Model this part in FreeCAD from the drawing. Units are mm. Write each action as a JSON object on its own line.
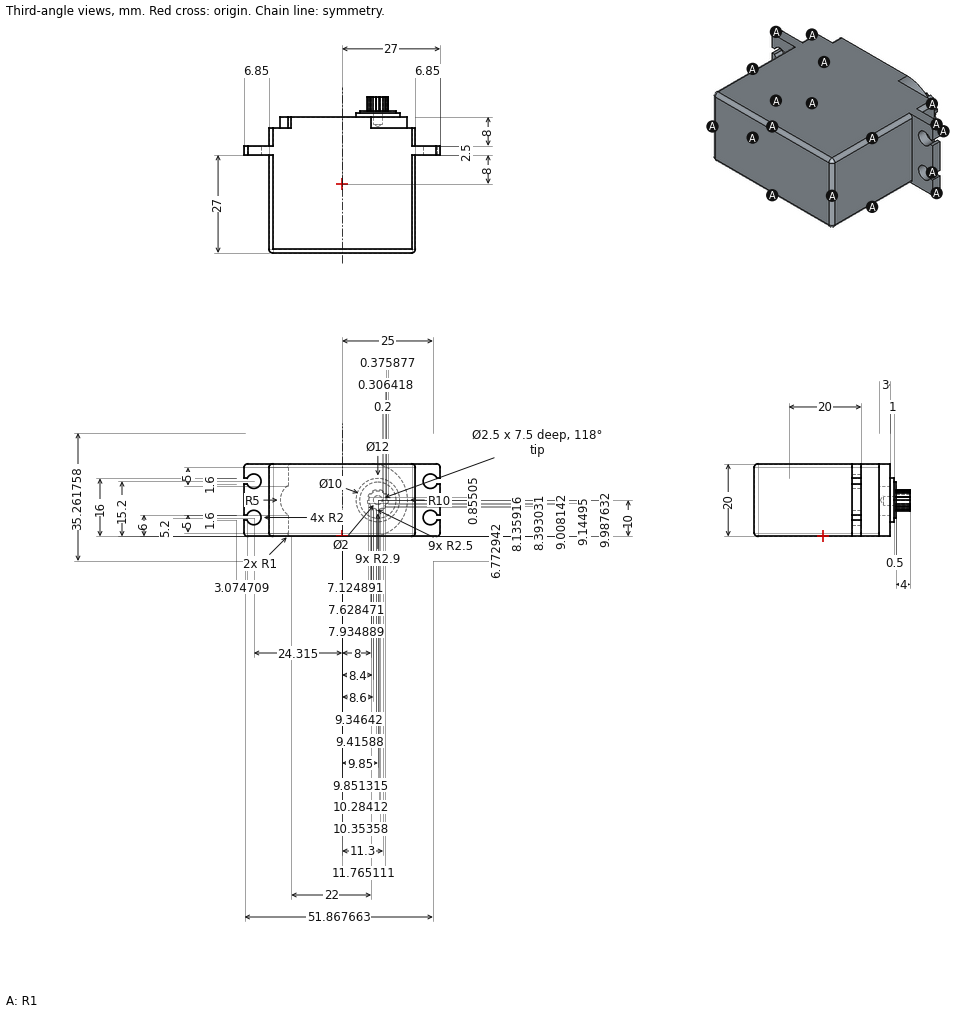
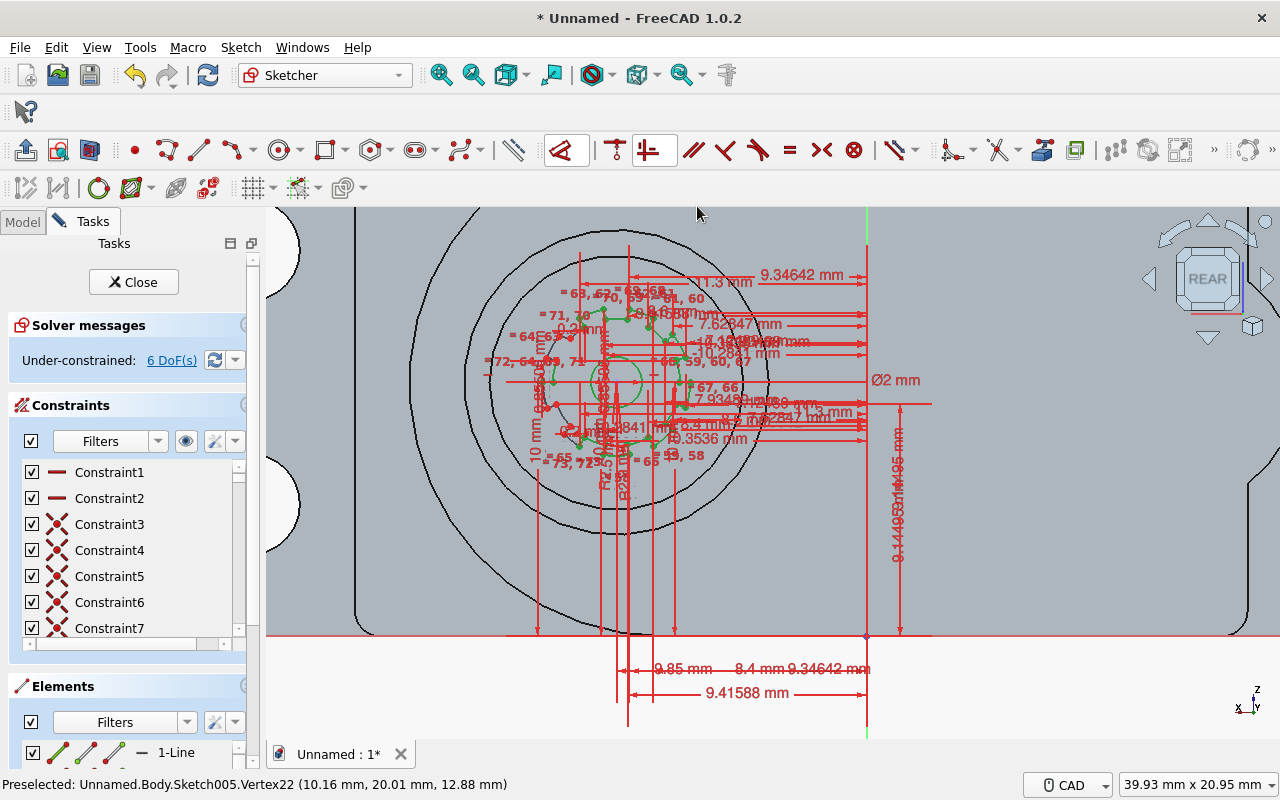
{"action": "left_click", "coordinate": [548, 408]}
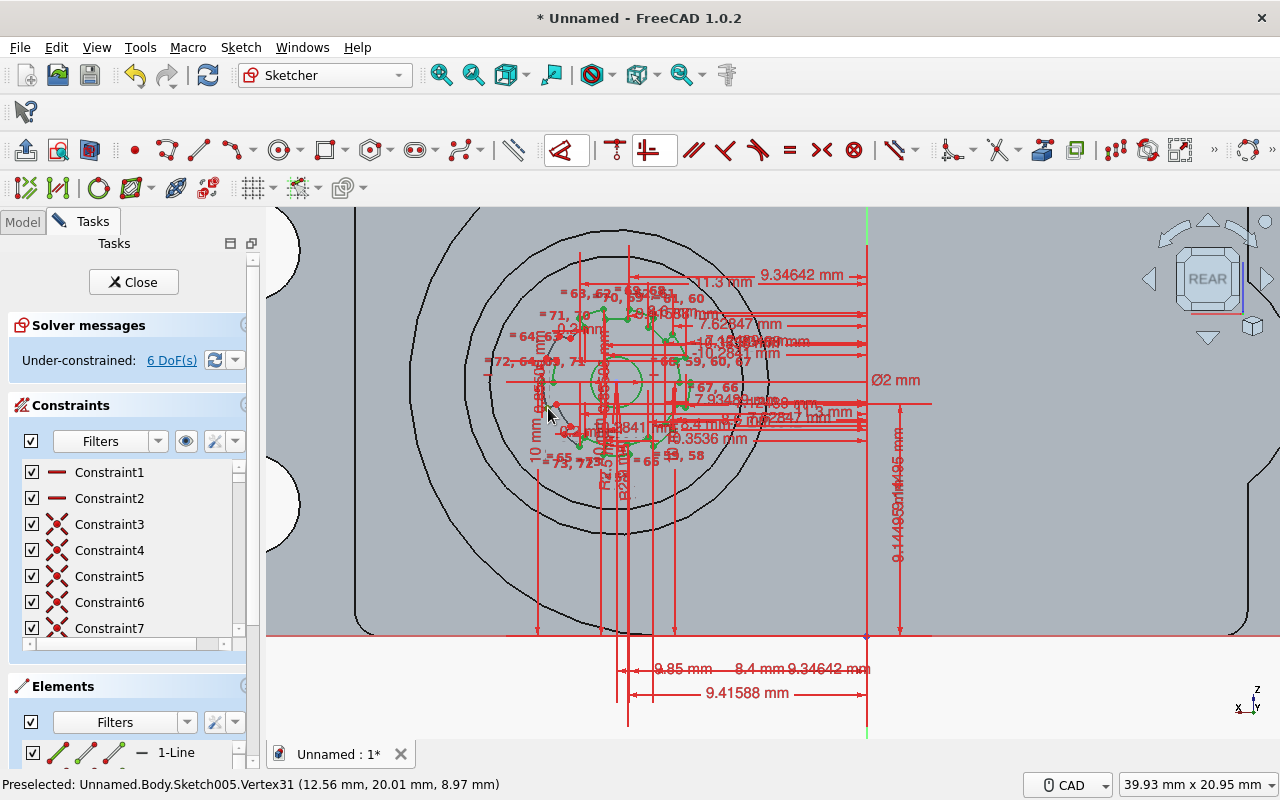
{"action": "left_click", "coordinate": [584, 150]}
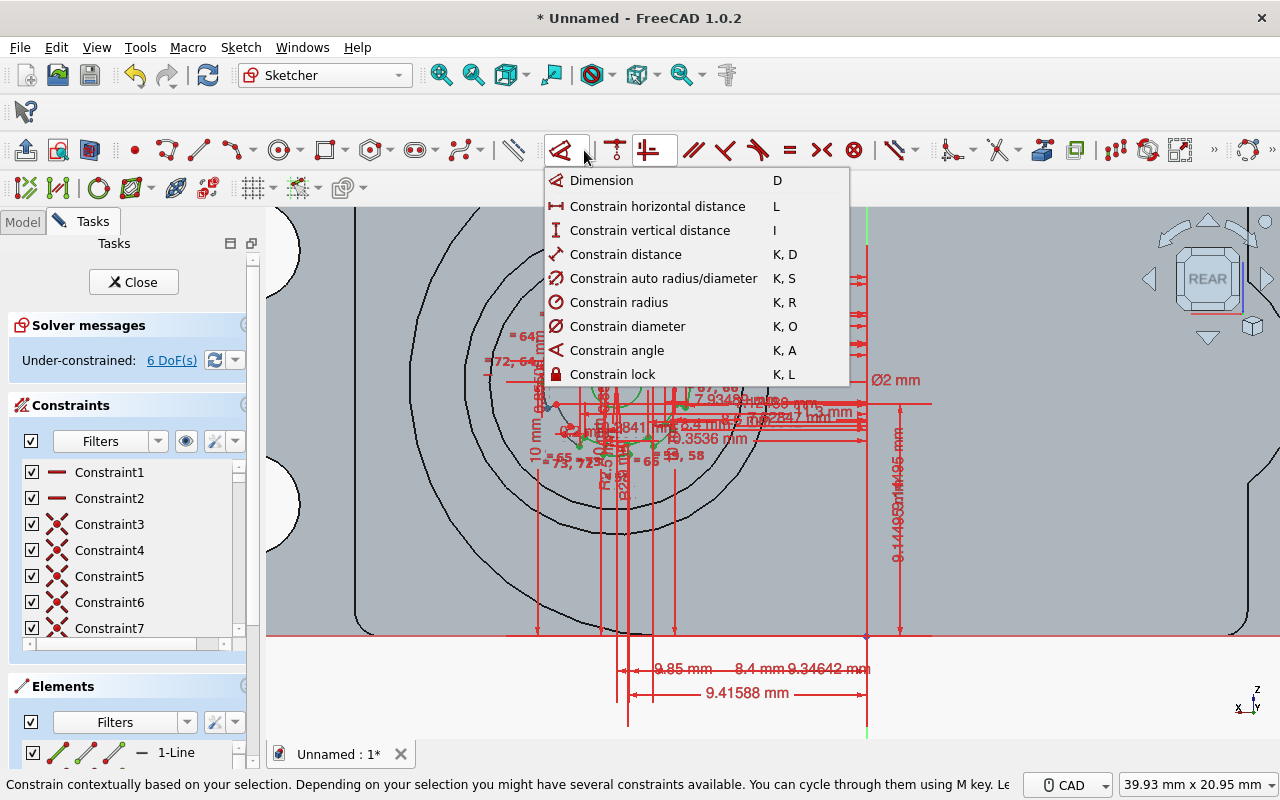
{"action": "left_click", "coordinate": [697, 230]}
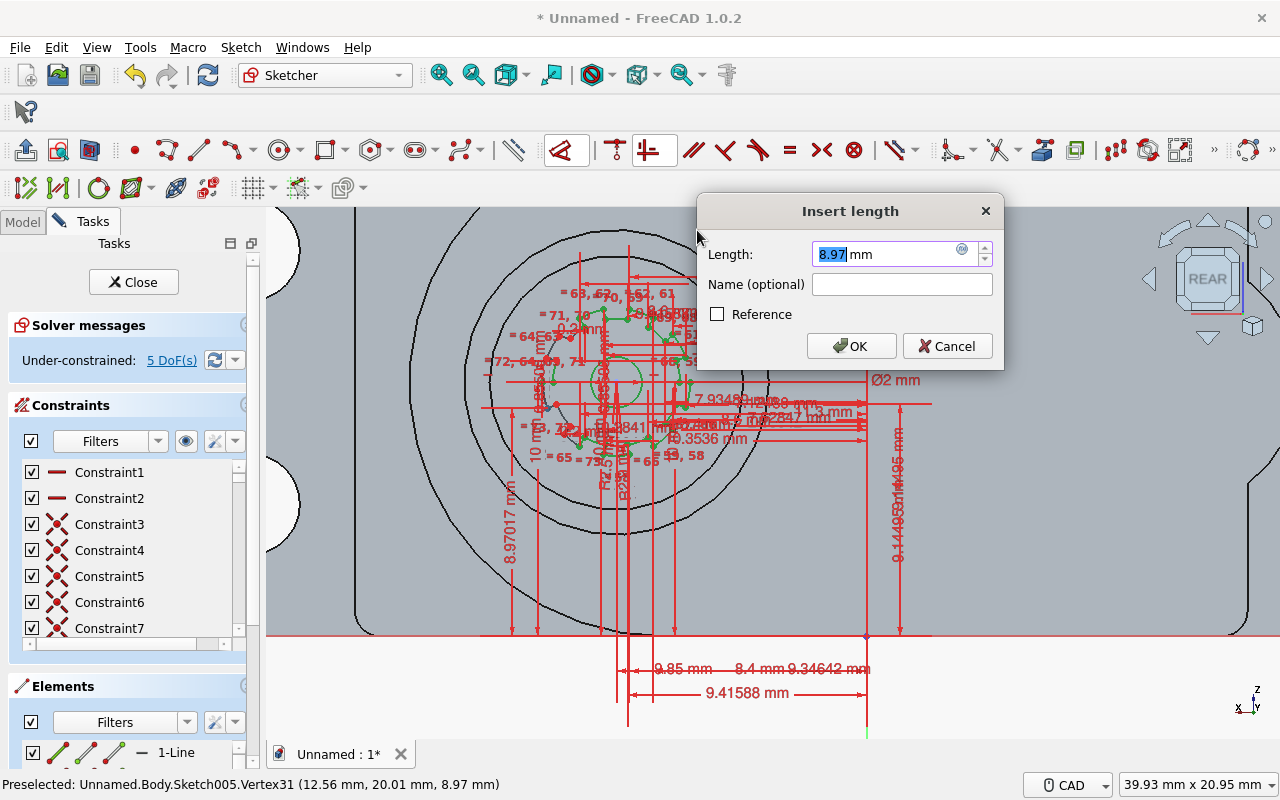
{"action": "type", "text": "9.008142"}
{"action": "key", "text": "Return"}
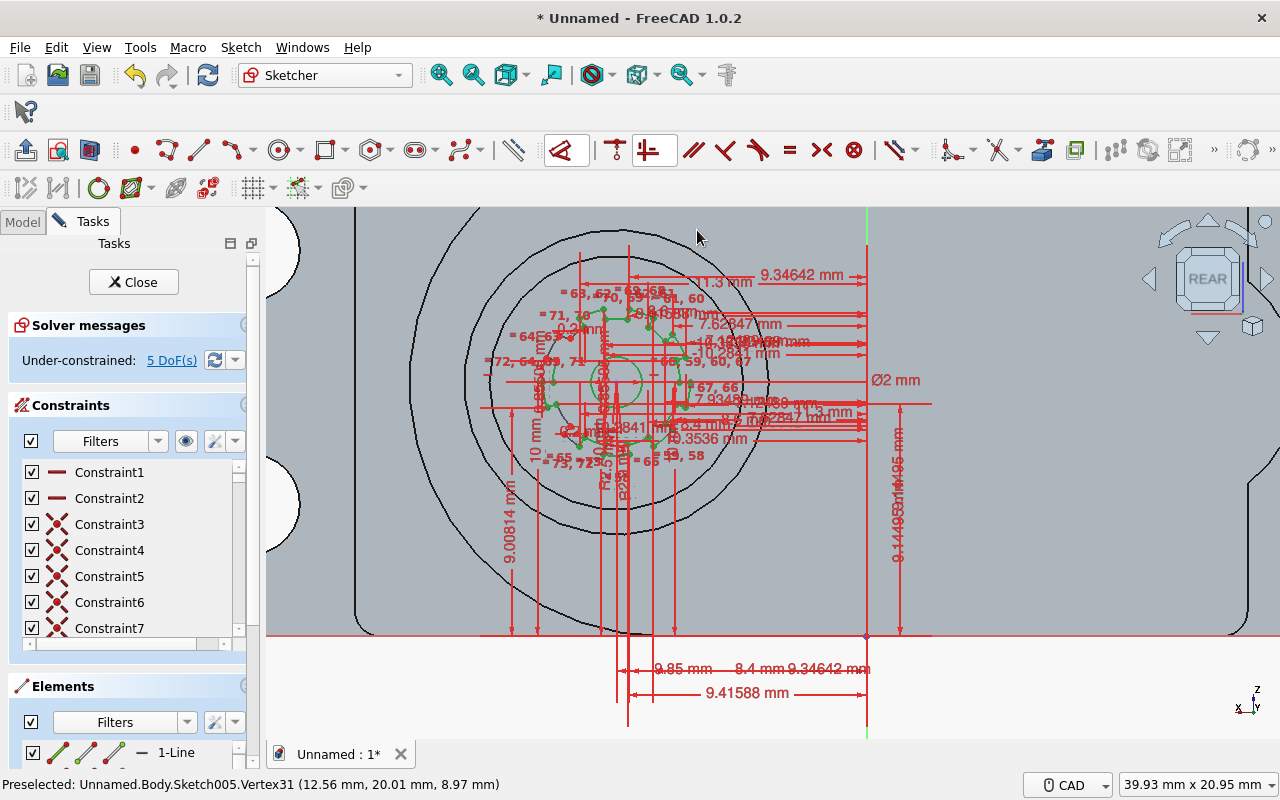
{"action": "left_click", "coordinate": [571, 426]}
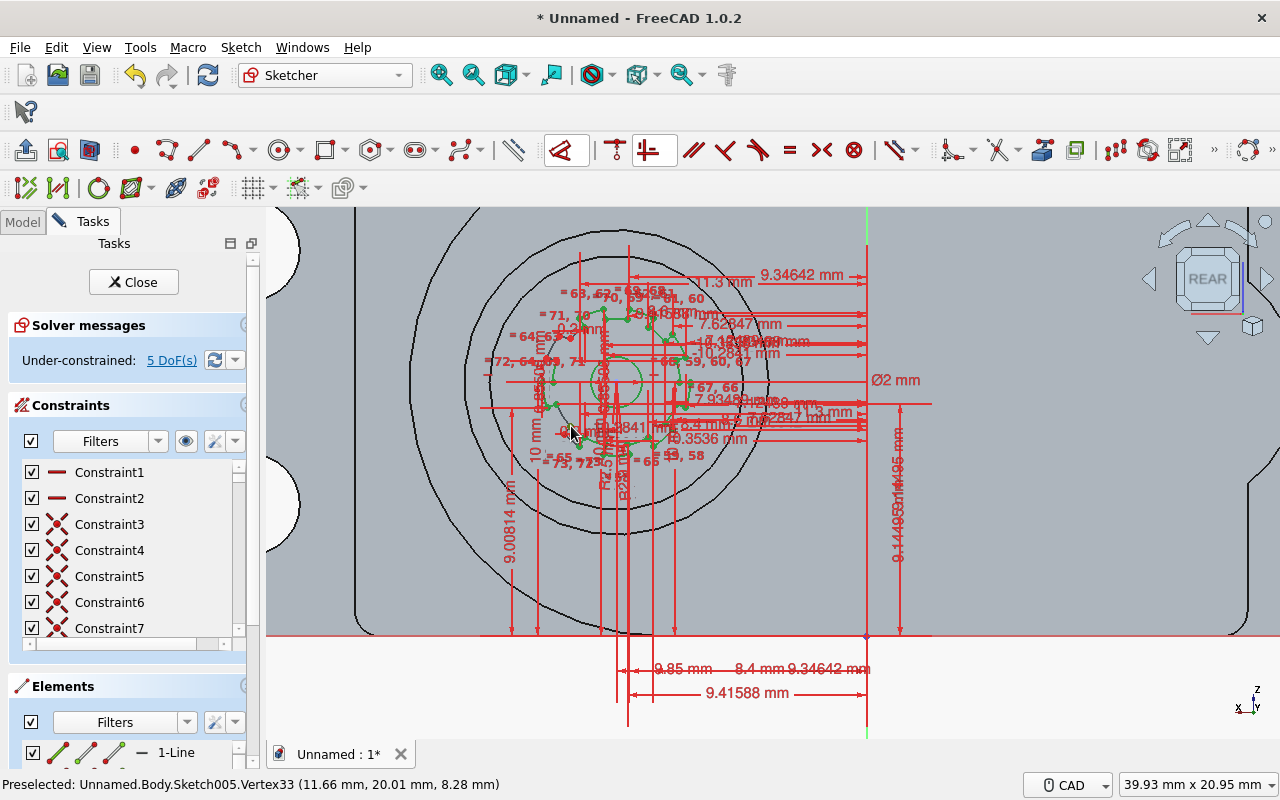
{"action": "key", "text": "i"}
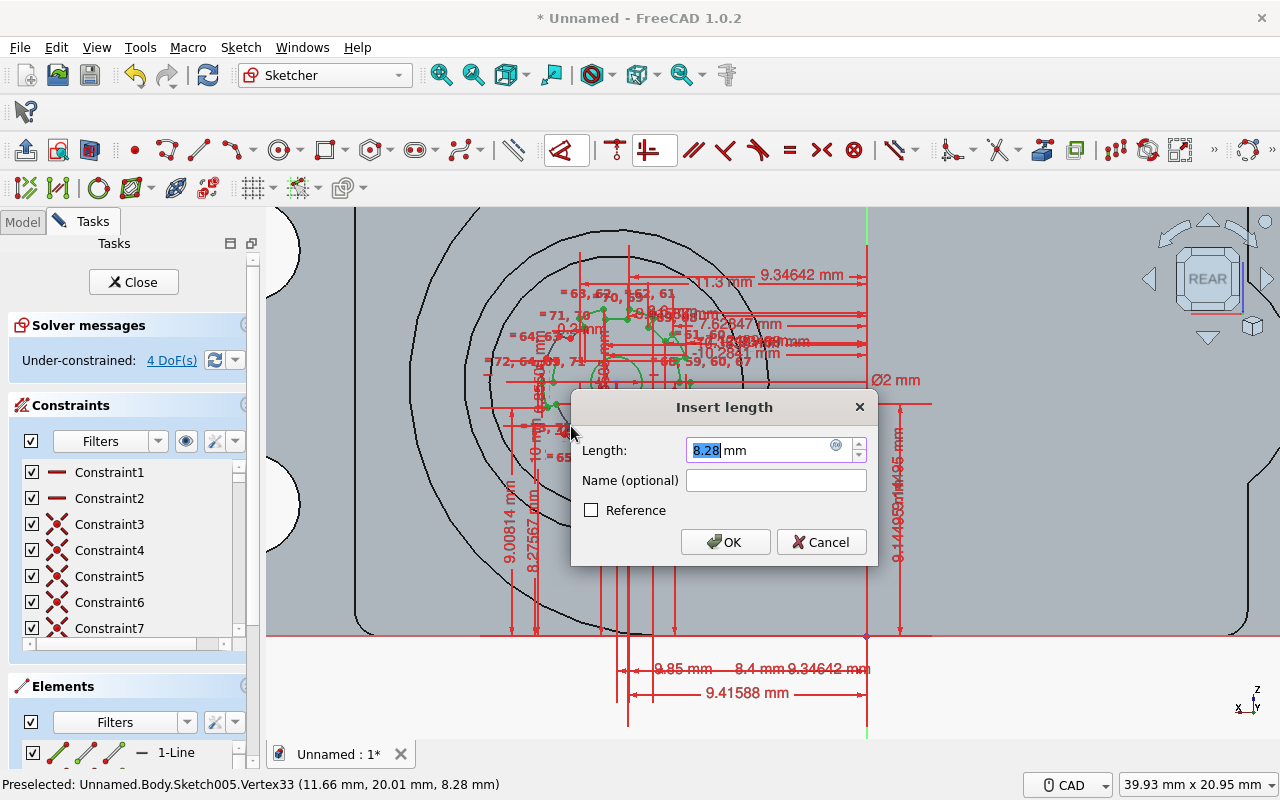
{"action": "type", "text": "8.393031"}
{"action": "key", "text": "Return"}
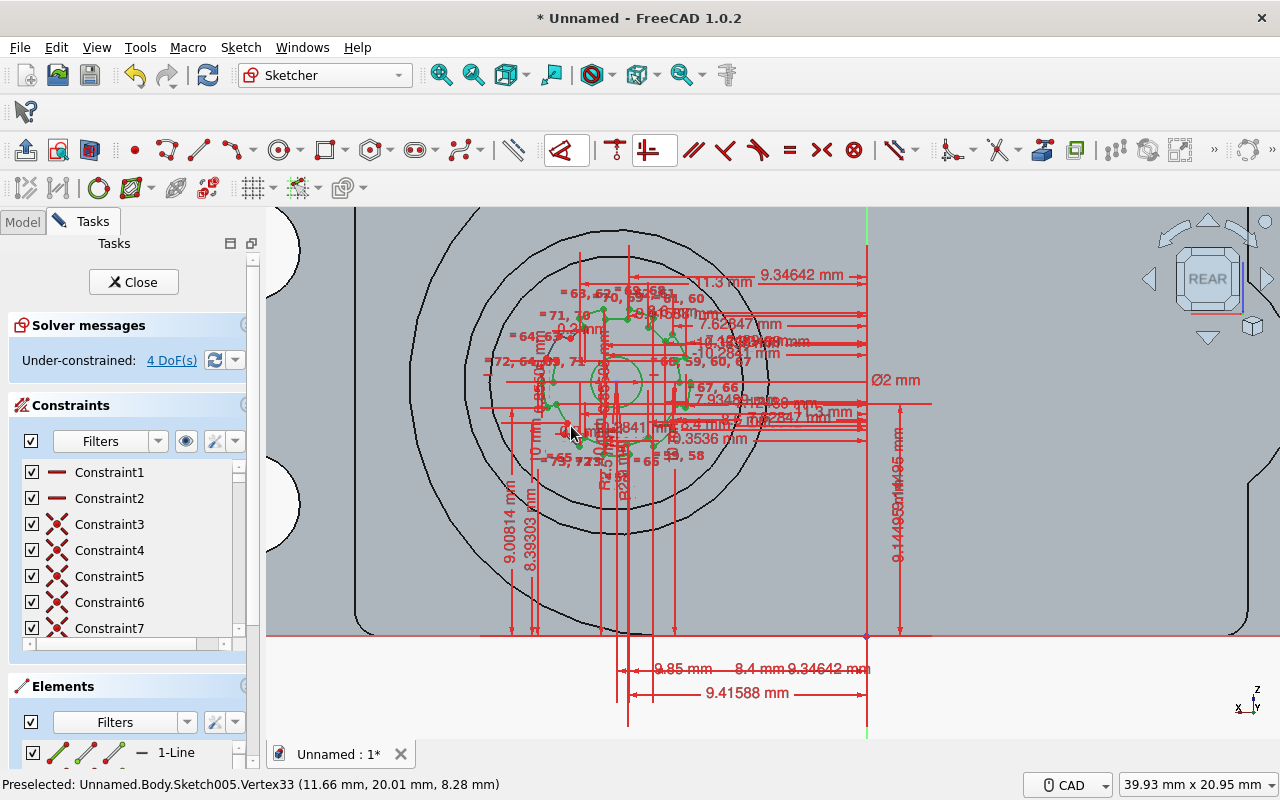
{"action": "left_click", "coordinate": [564, 434]}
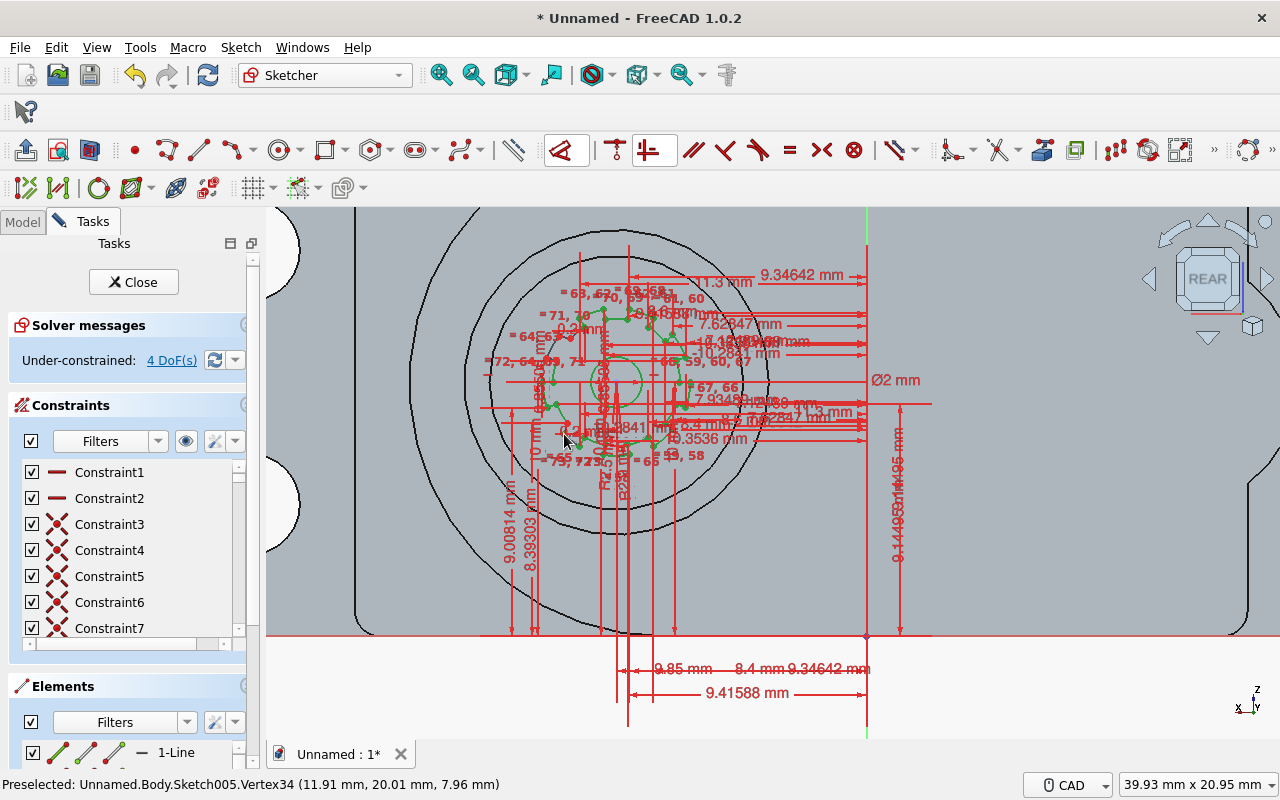
{"action": "left_click", "coordinate": [584, 150]}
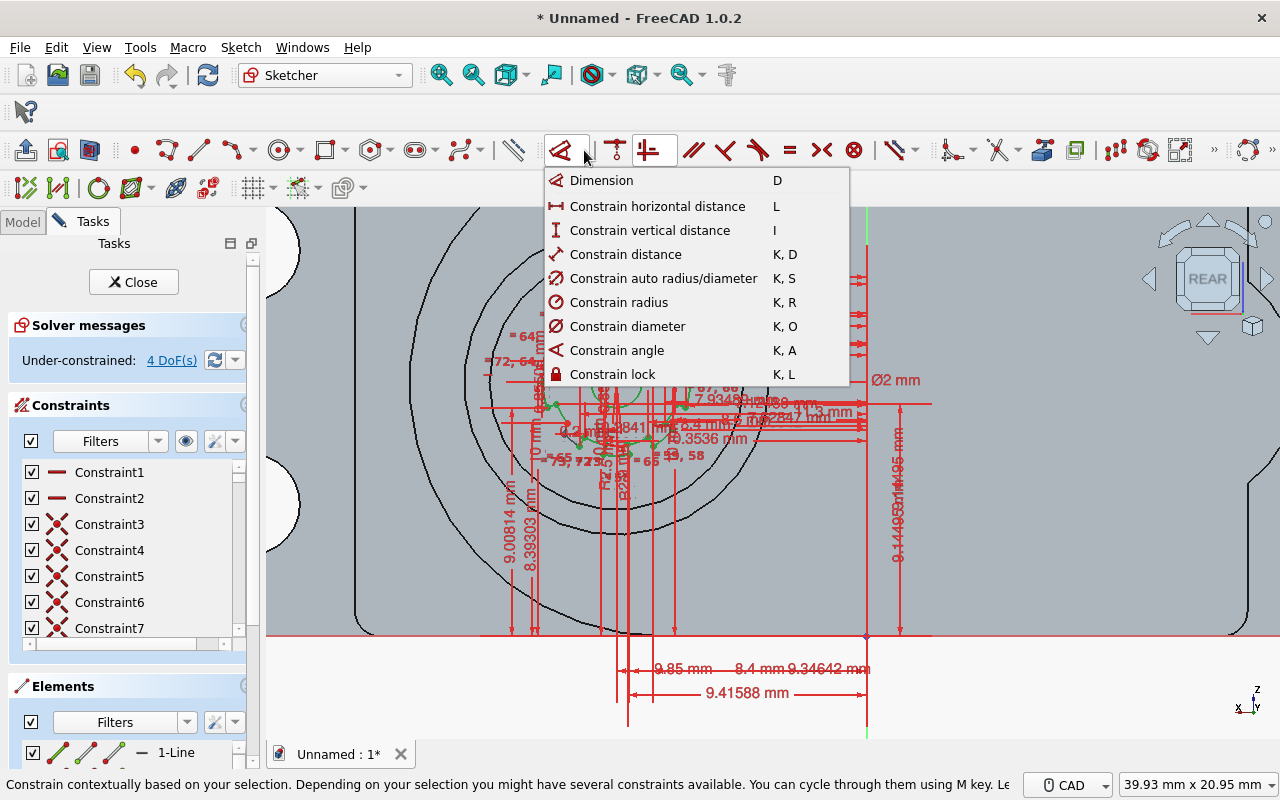
{"action": "left_click", "coordinate": [697, 230]}